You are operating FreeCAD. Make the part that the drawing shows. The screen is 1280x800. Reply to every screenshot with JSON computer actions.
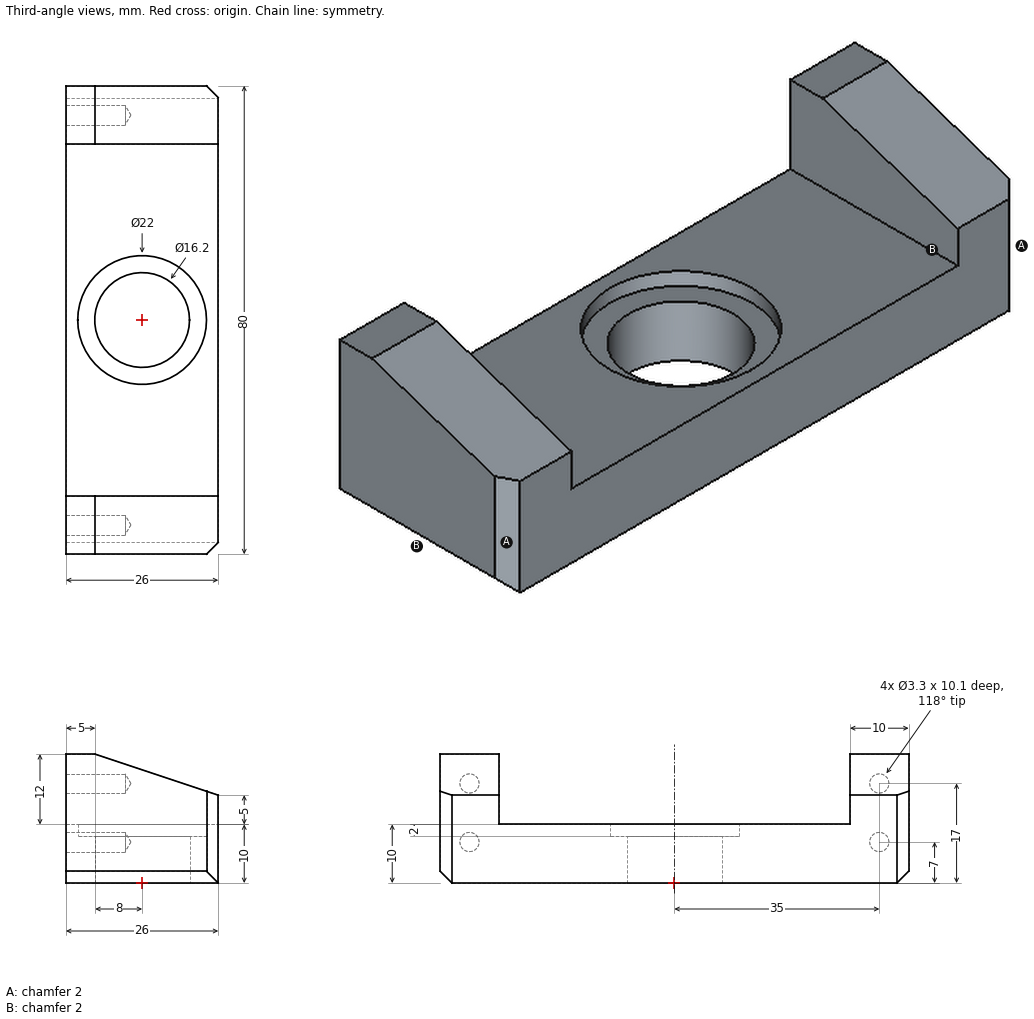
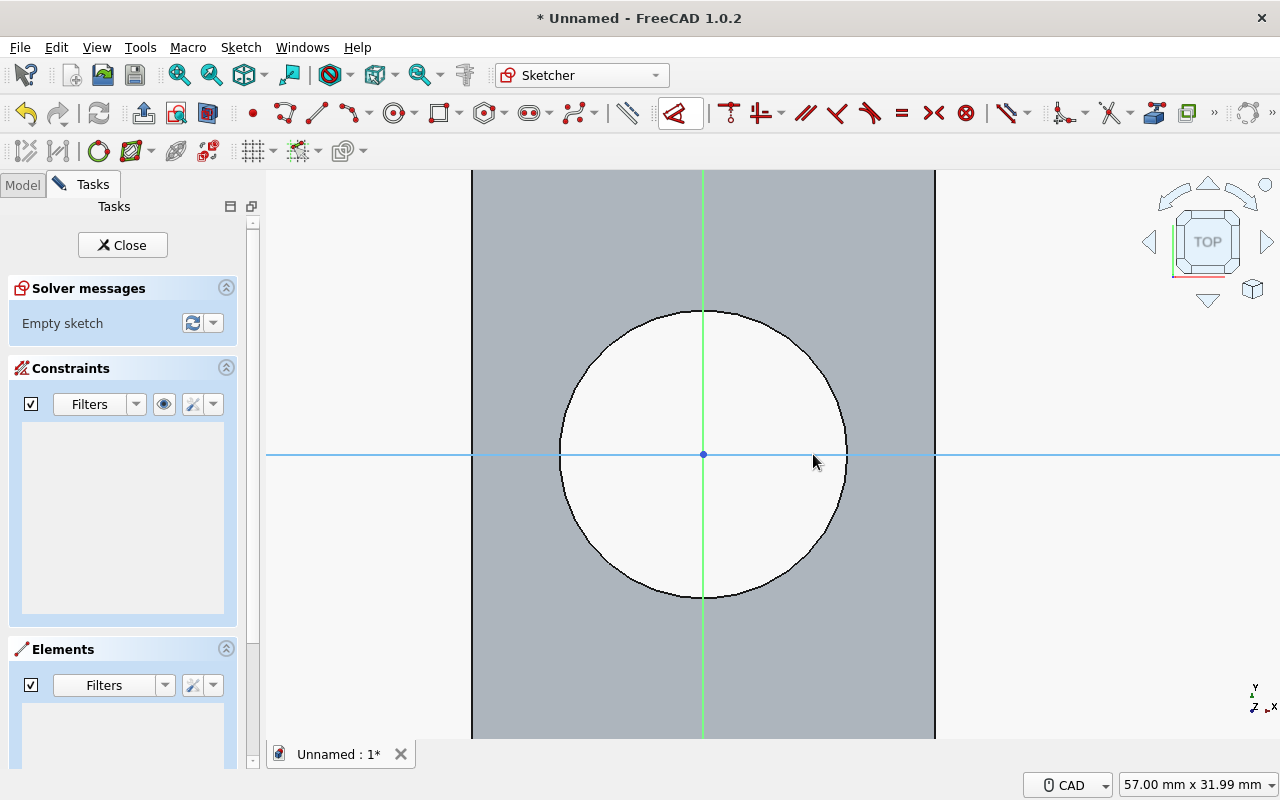
{"action": "left_click", "coordinate": [394, 114]}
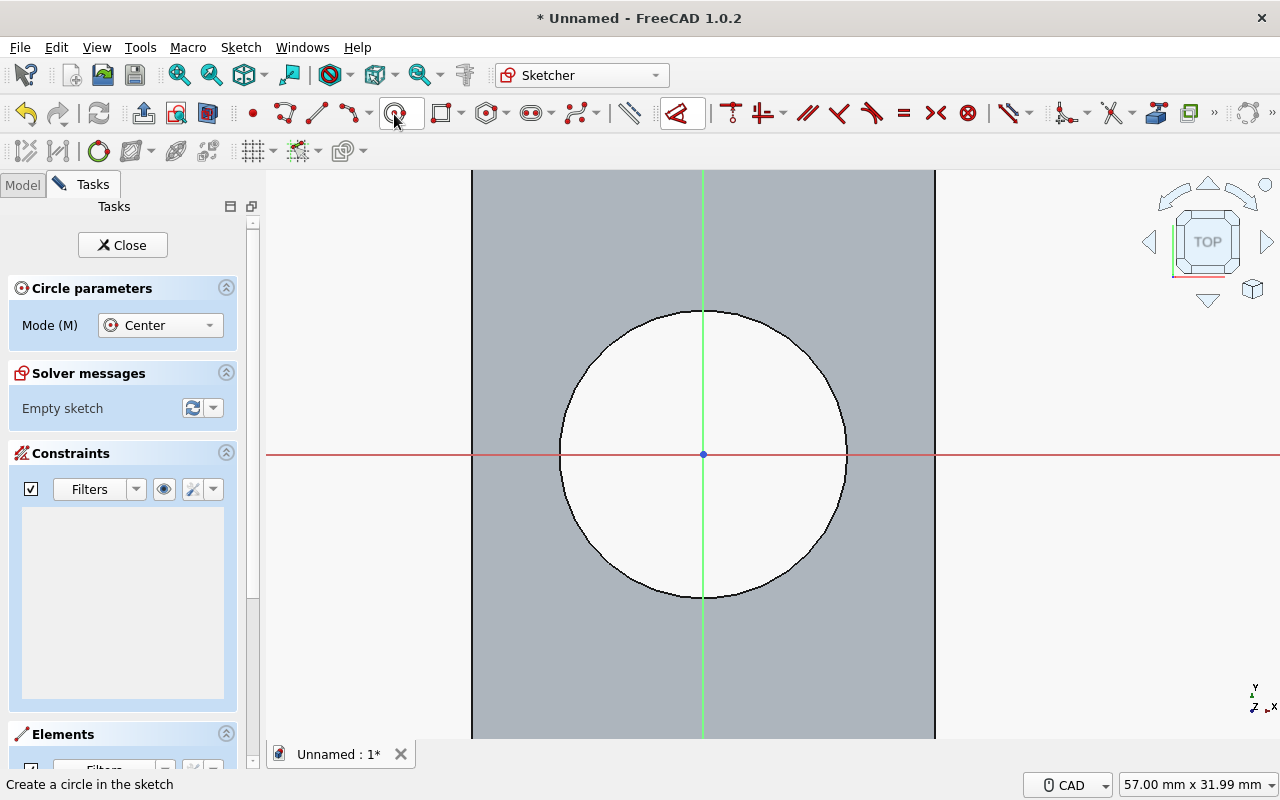
{"action": "left_click", "coordinate": [703, 454]}
{"action": "left_click", "coordinate": [842, 316]}
{"action": "key", "text": "Escape"}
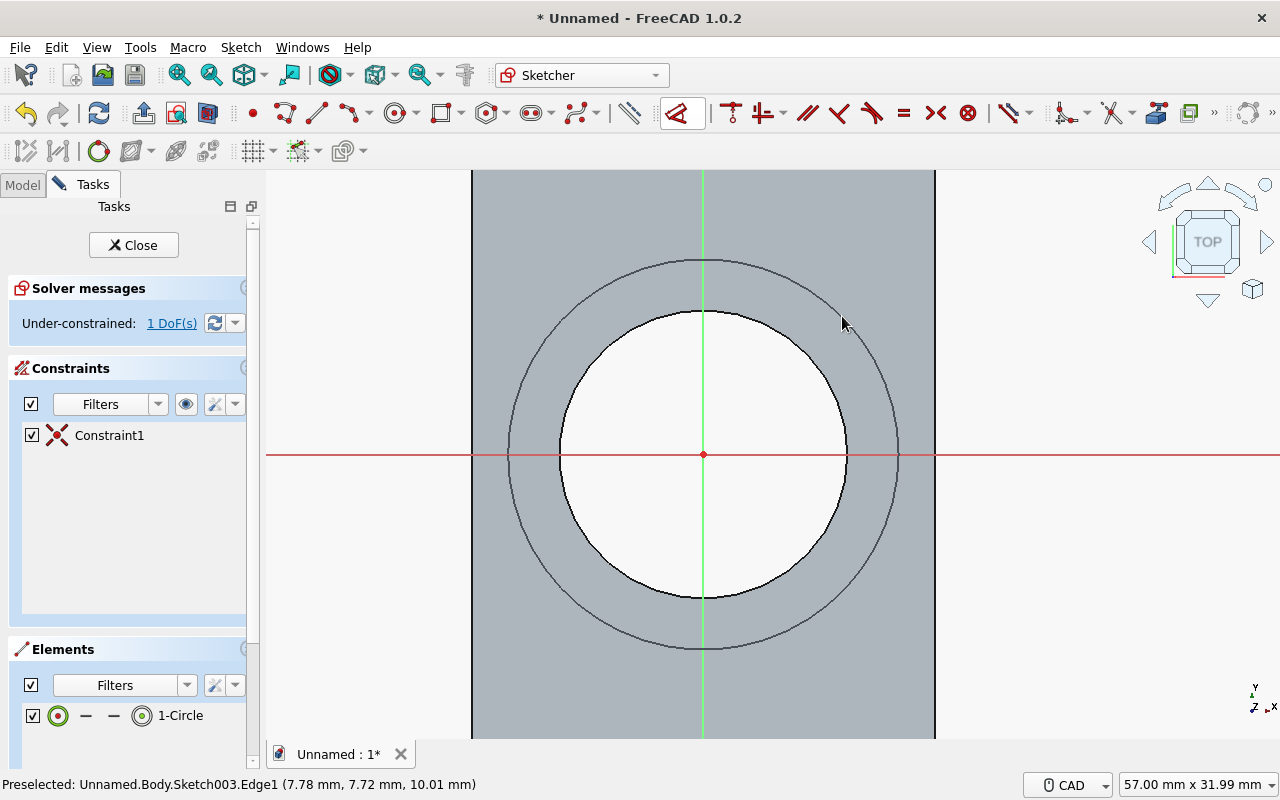
{"action": "left_click", "coordinate": [841, 316]}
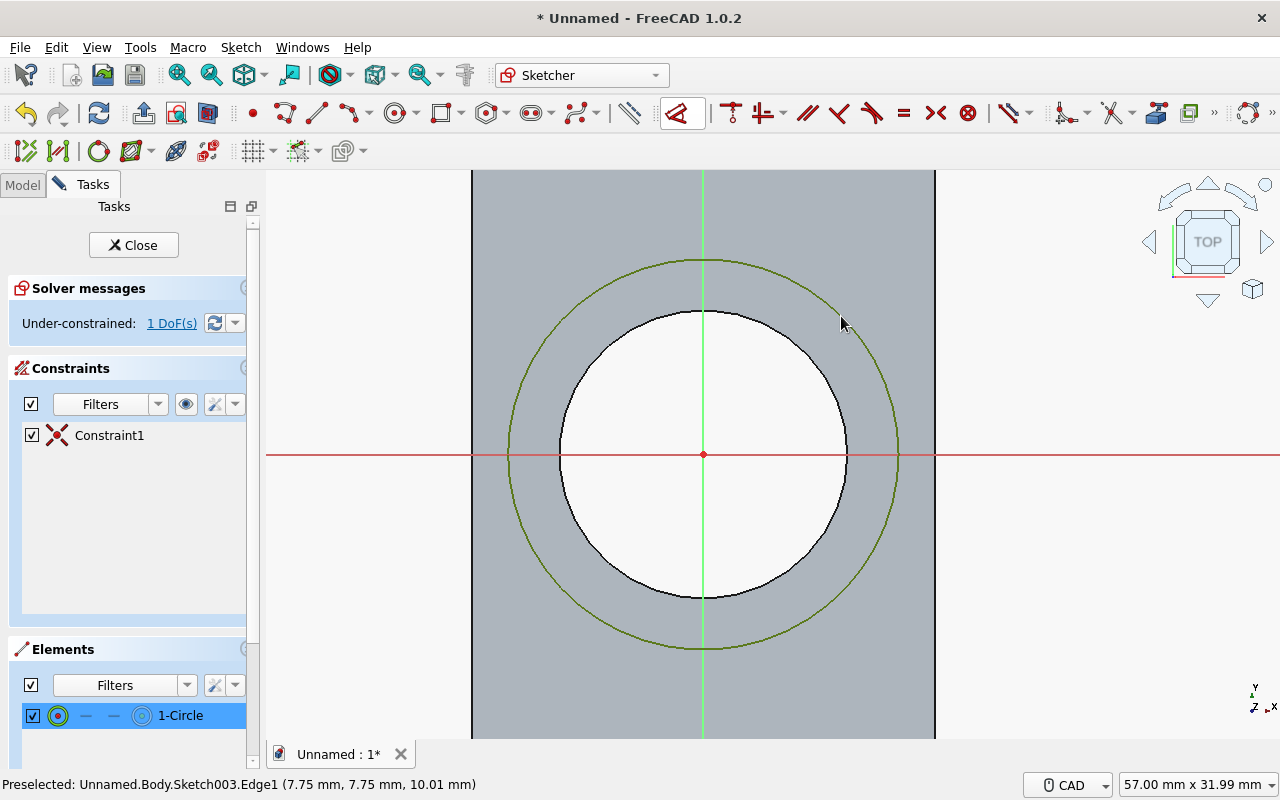
{"action": "left_click", "coordinate": [700, 114]}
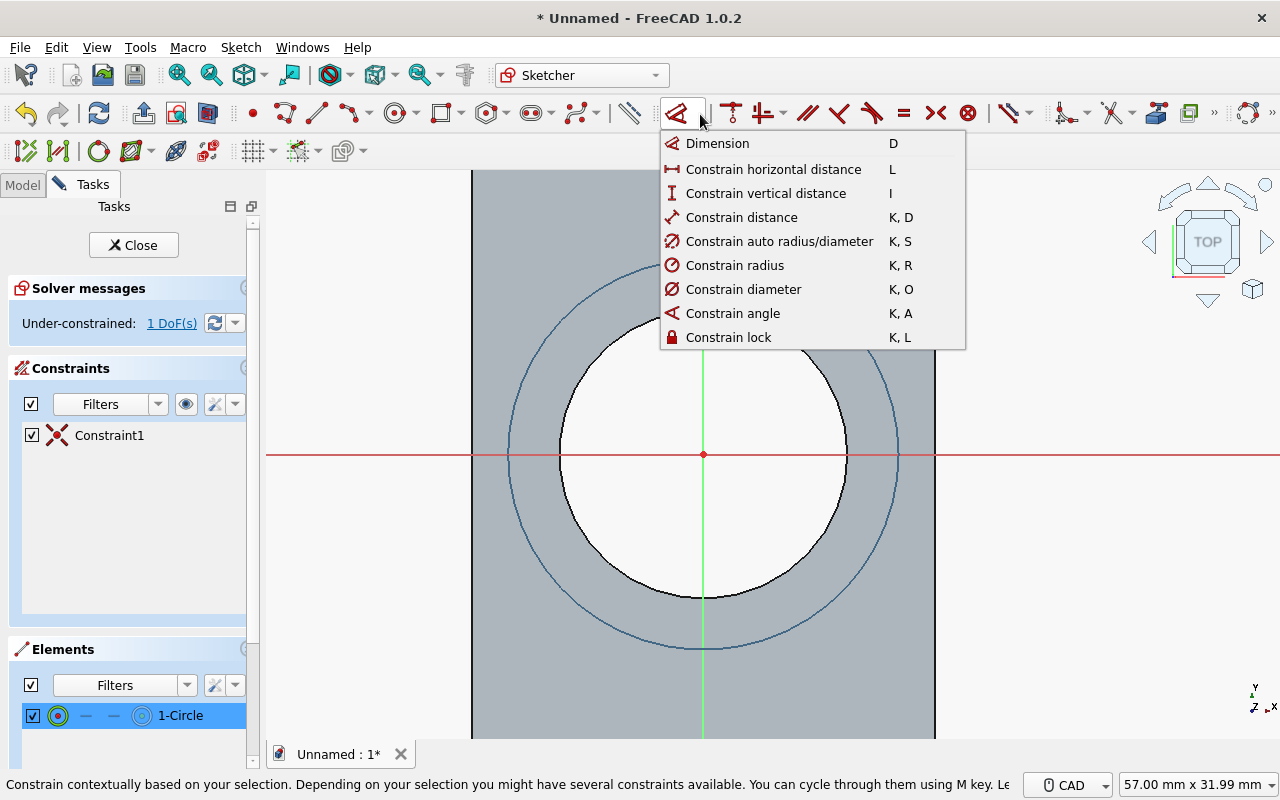
{"action": "left_click", "coordinate": [813, 289]}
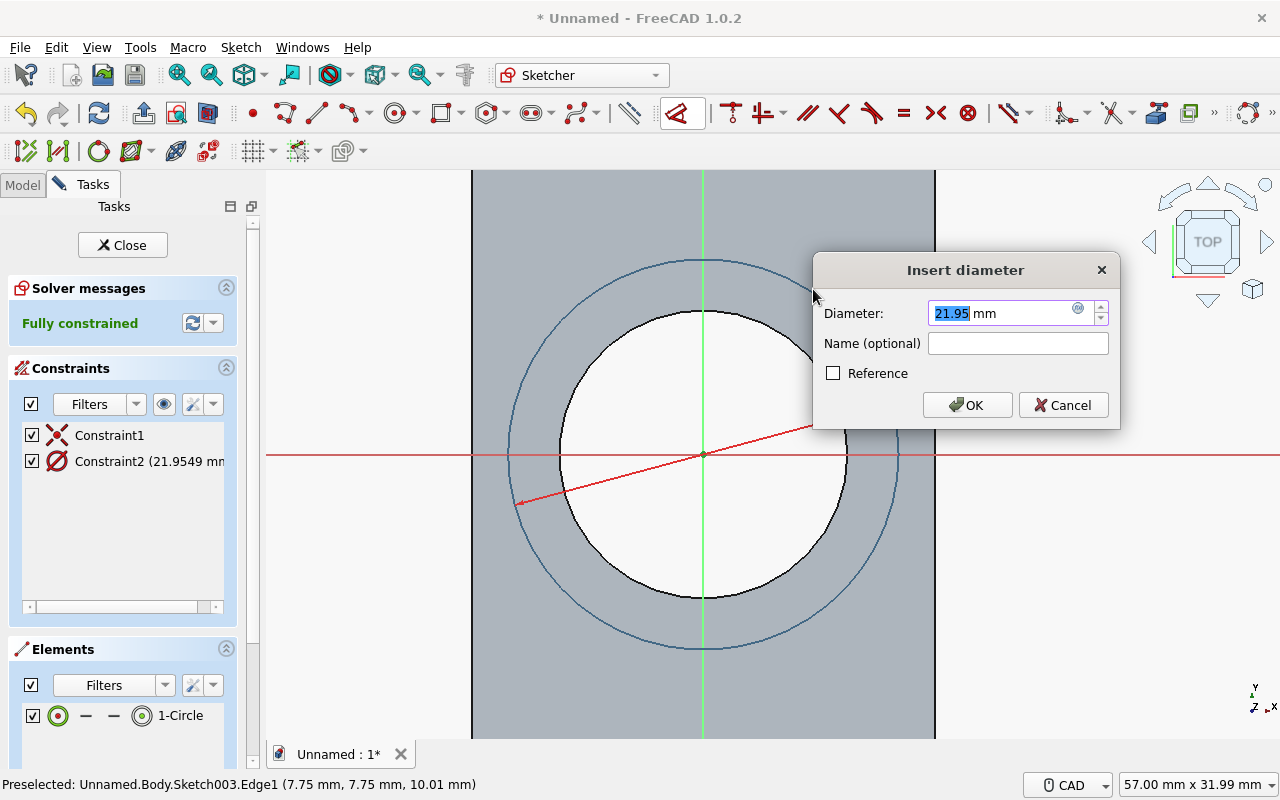
{"action": "type", "text": "22"}
{"action": "key", "text": "Return"}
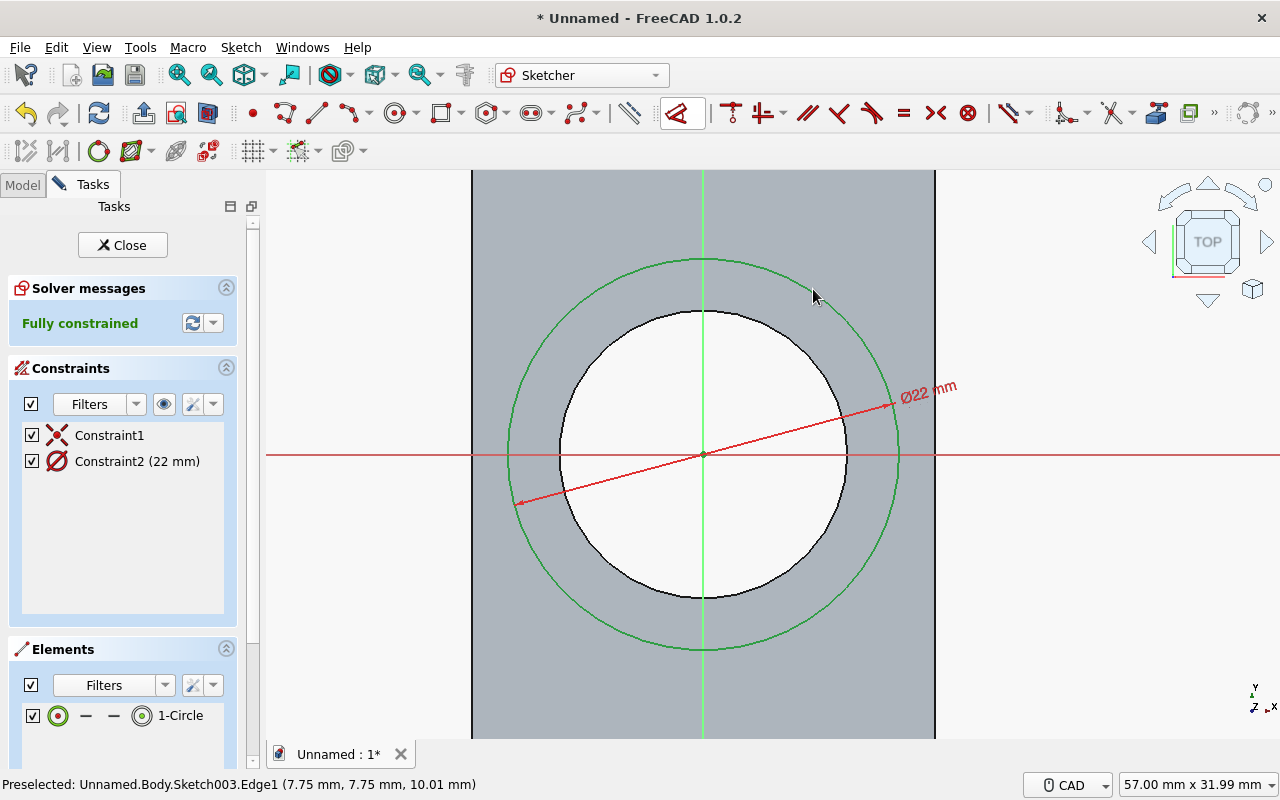
{"action": "left_click", "coordinate": [123, 245]}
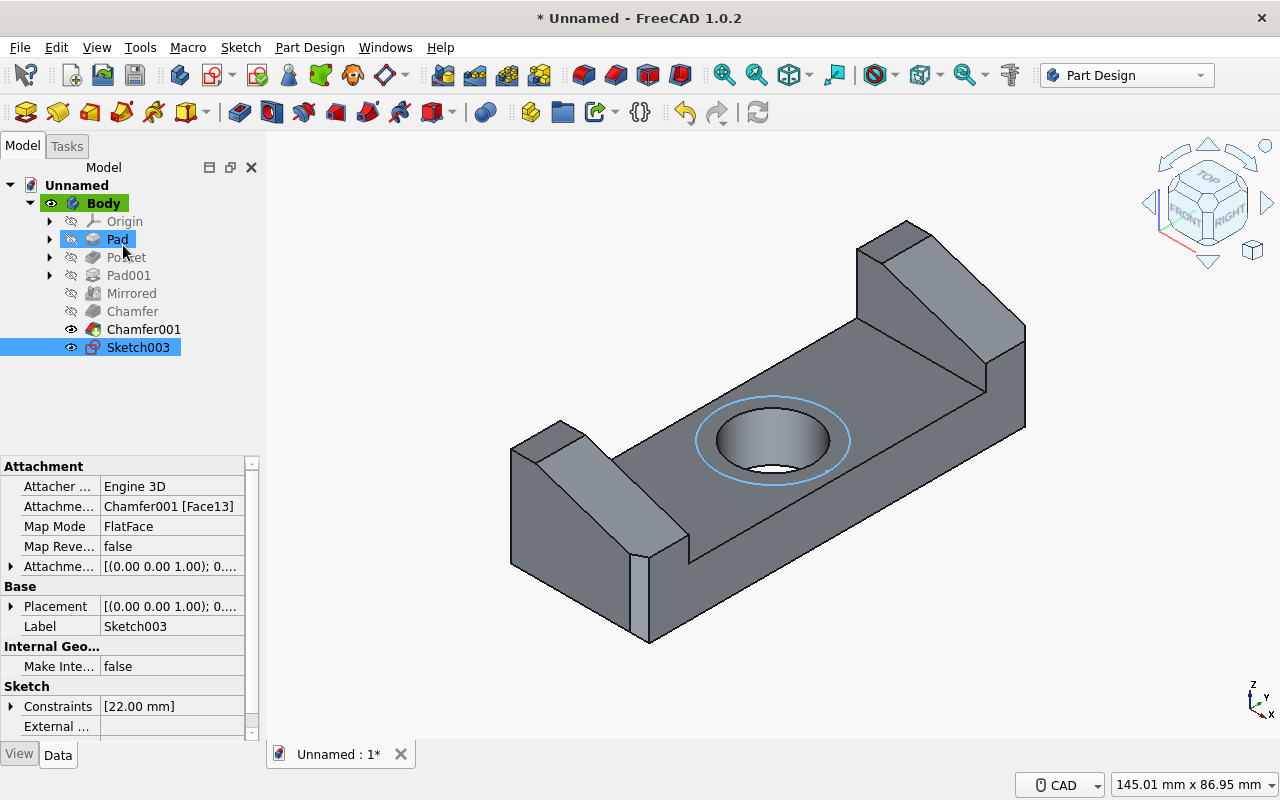
{"action": "left_click", "coordinate": [240, 112]}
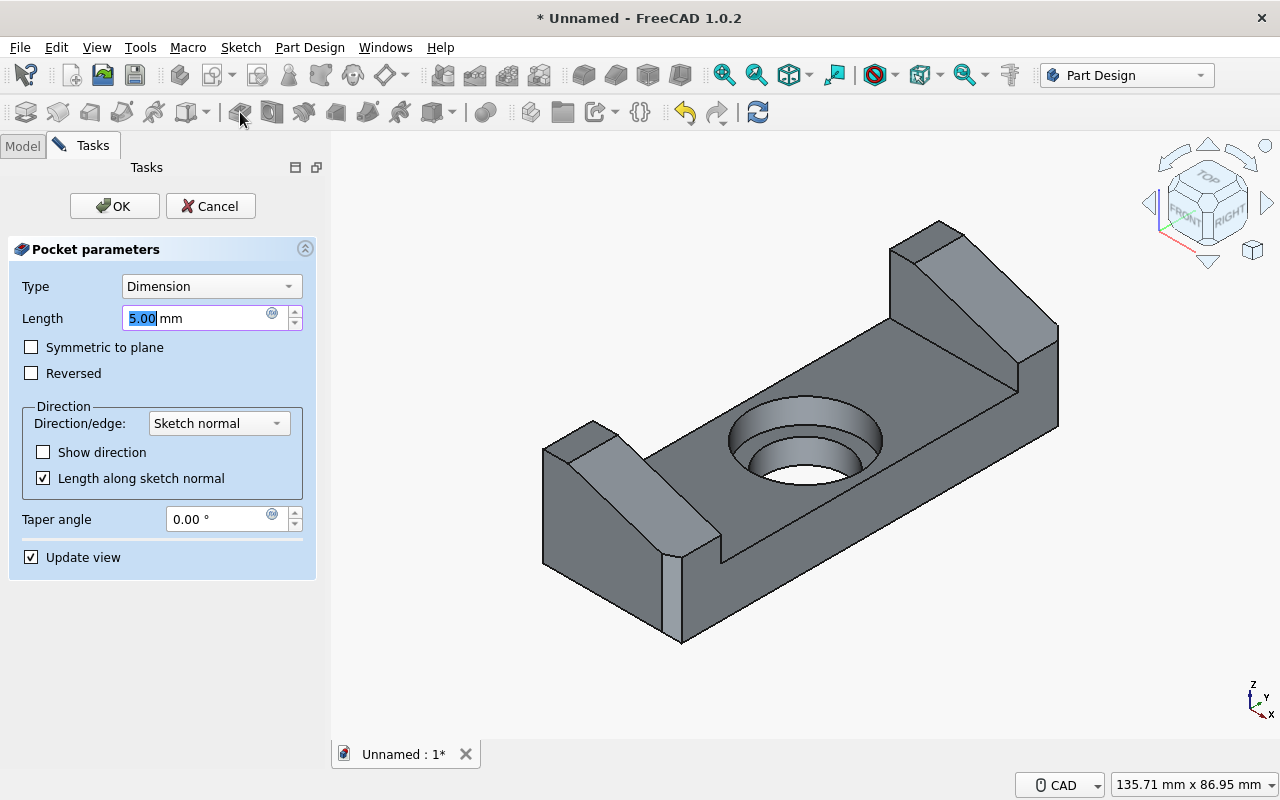
{"action": "type", "text": "2"}
{"action": "key", "text": "Tab"}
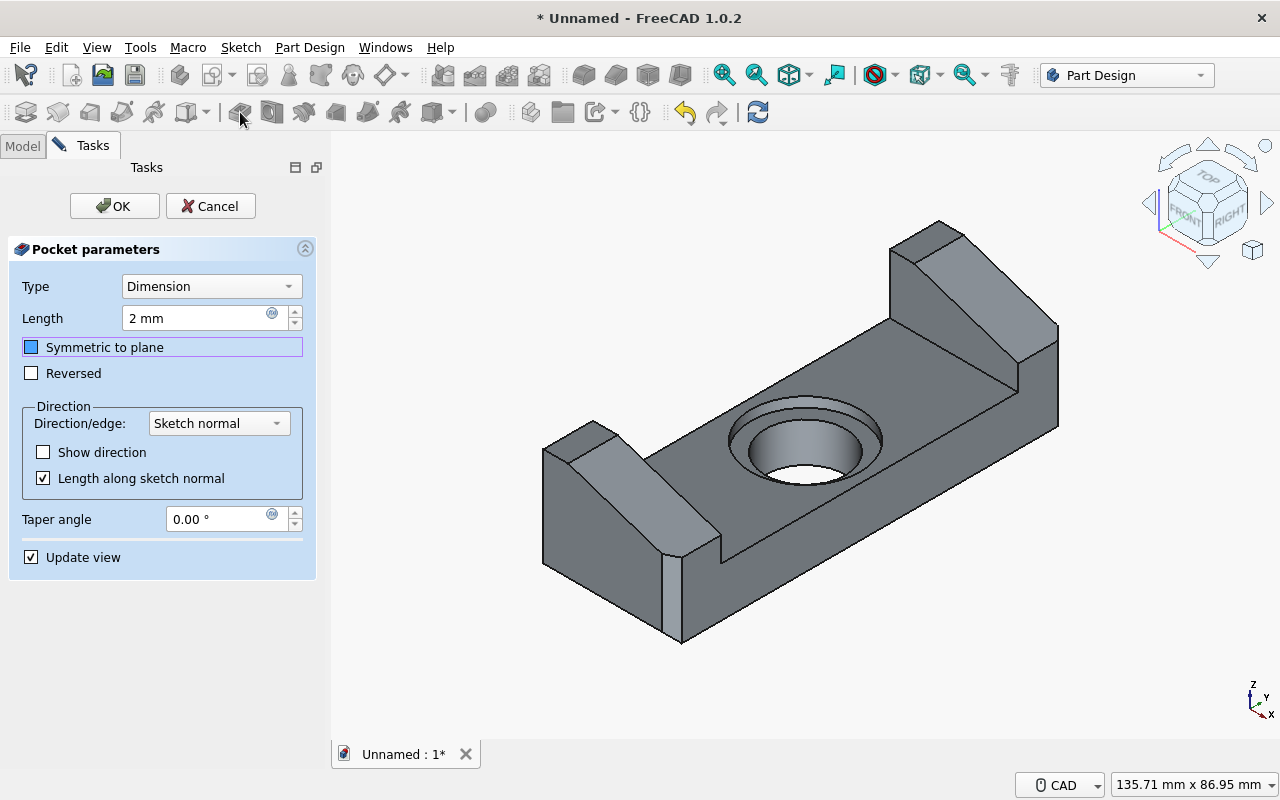
{"action": "left_click", "coordinate": [115, 206]}